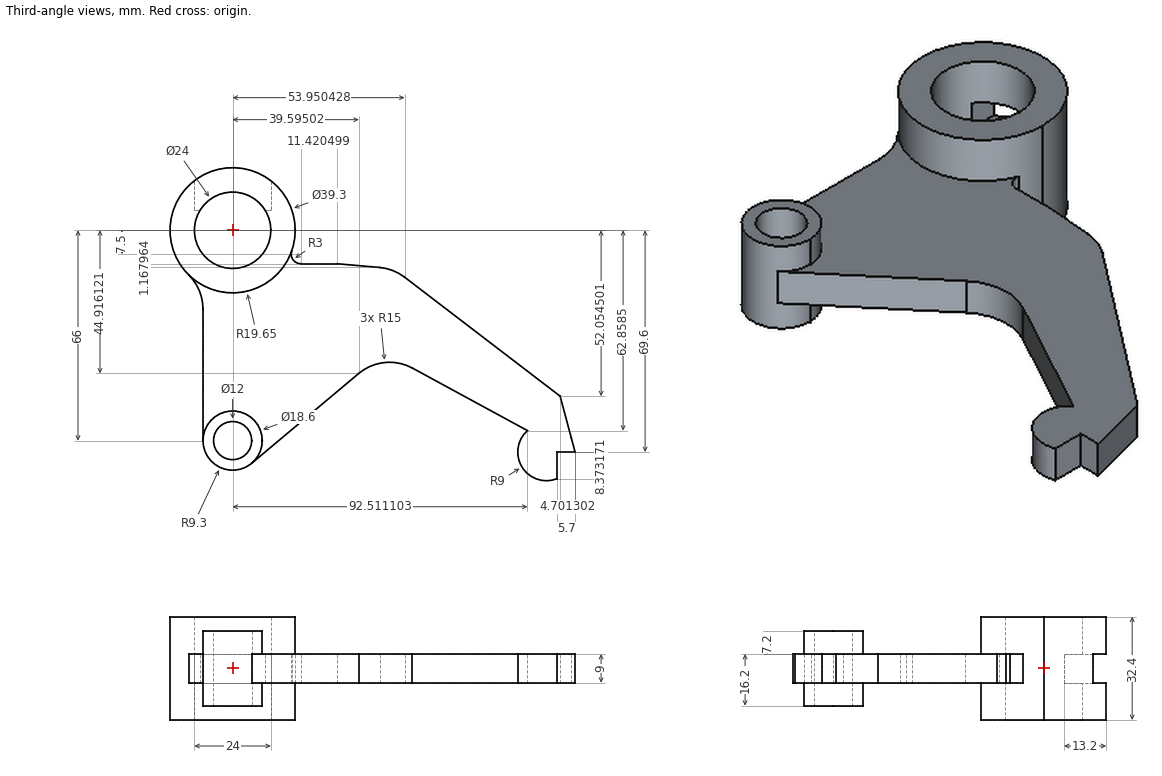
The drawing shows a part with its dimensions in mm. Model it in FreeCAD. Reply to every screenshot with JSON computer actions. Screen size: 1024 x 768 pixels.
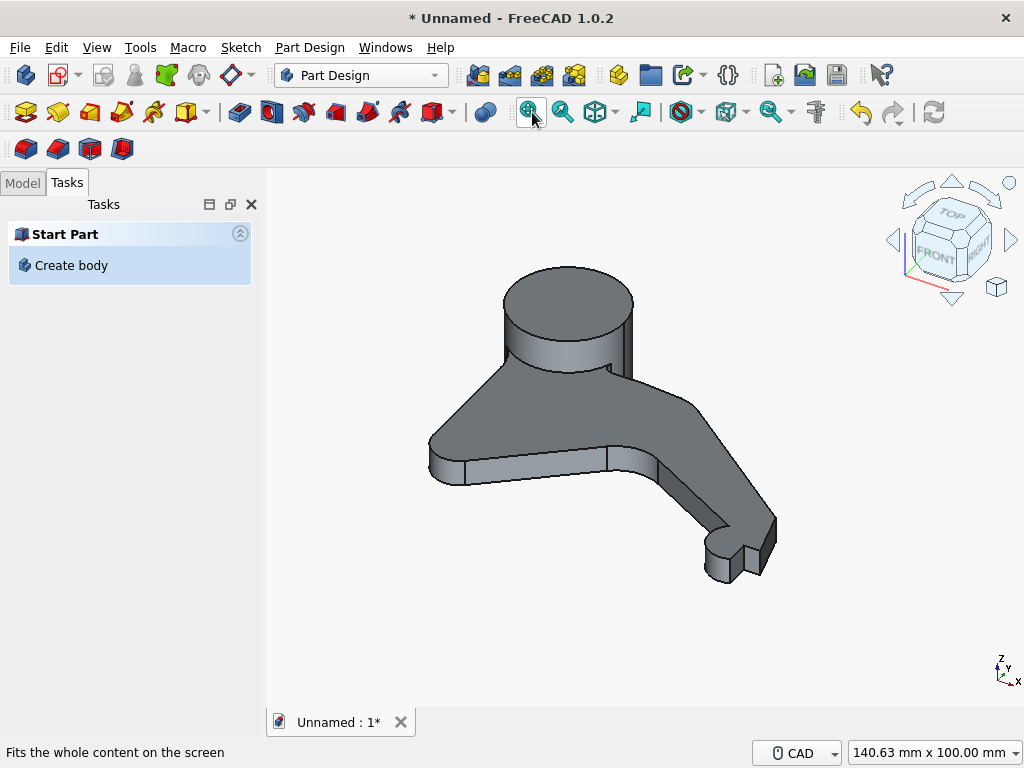
{"action": "left_click", "coordinate": [533, 416]}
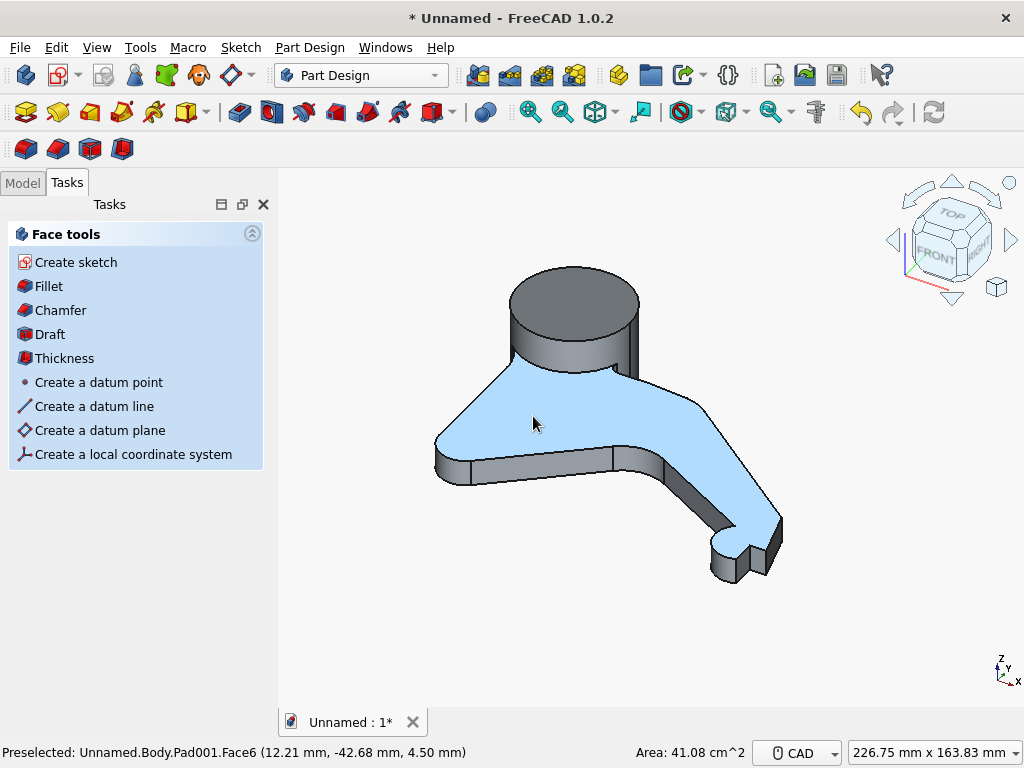
{"action": "left_click", "coordinate": [58, 76]}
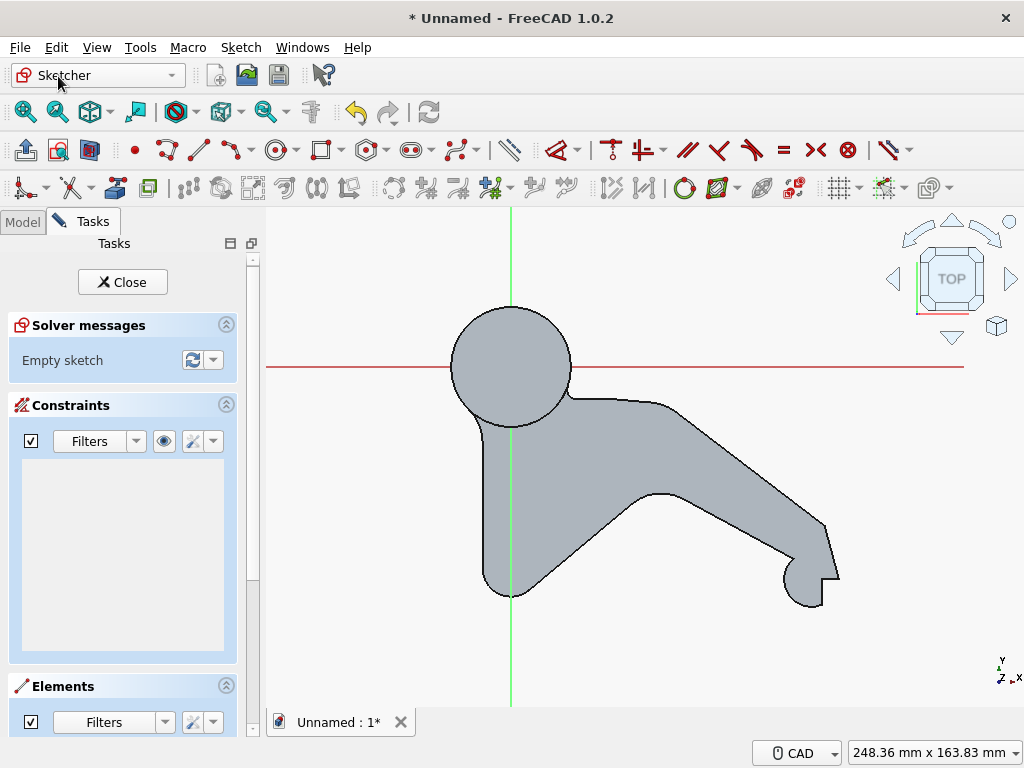
{"action": "left_click", "coordinate": [90, 150]}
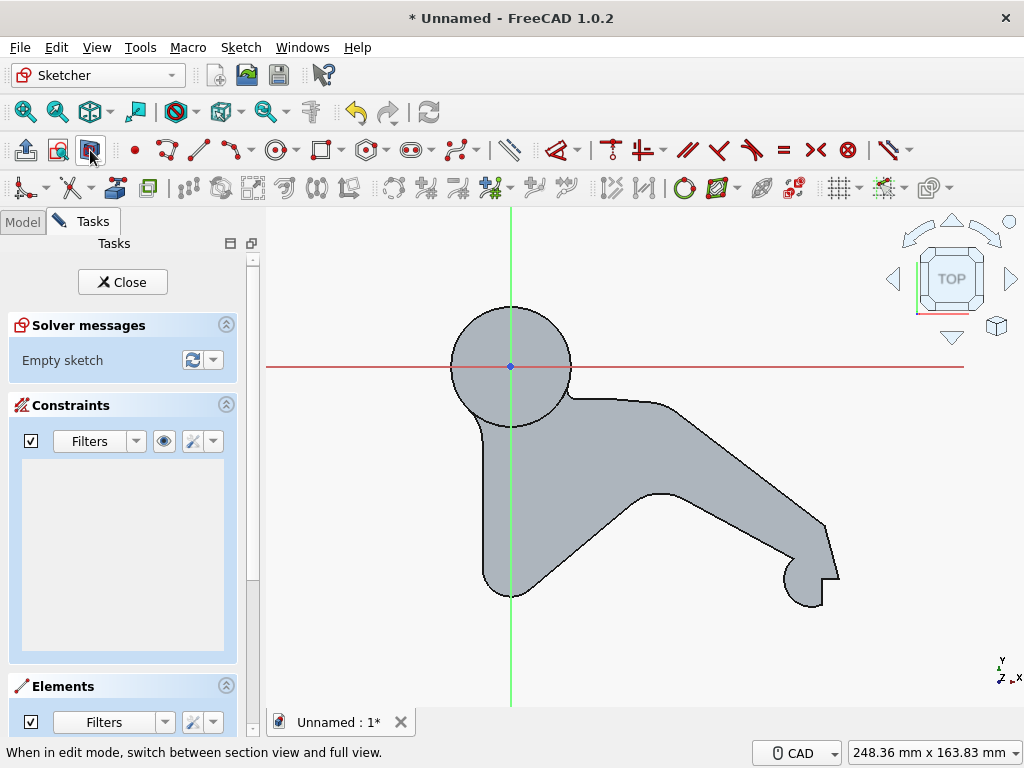
{"action": "scroll", "coordinate": [498, 590], "scroll_direction": "up", "scroll_amount": 9}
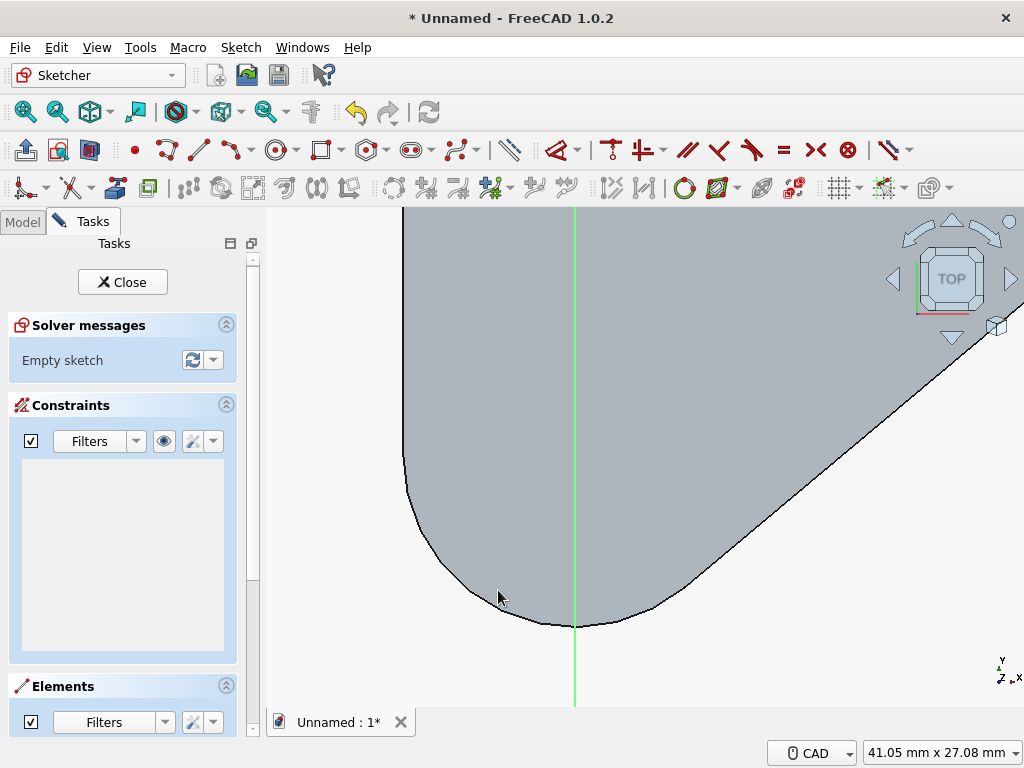
{"action": "left_click", "coordinate": [276, 150]}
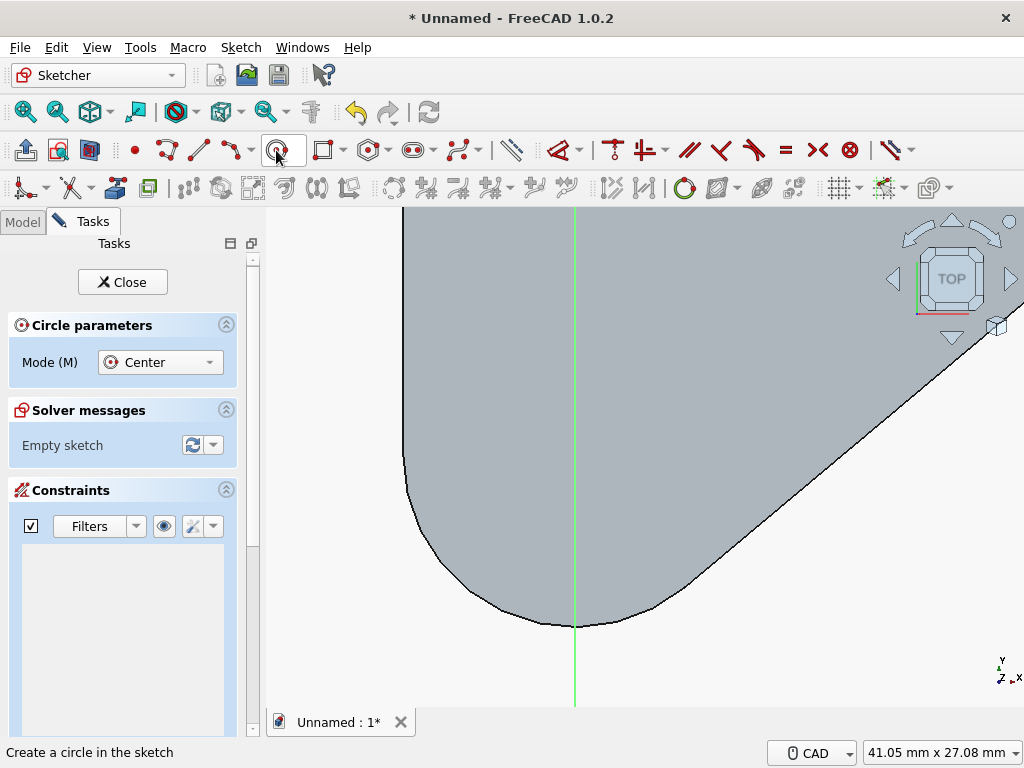
{"action": "left_click", "coordinate": [575, 455]}
{"action": "mouse_move", "coordinate": [696, 334]}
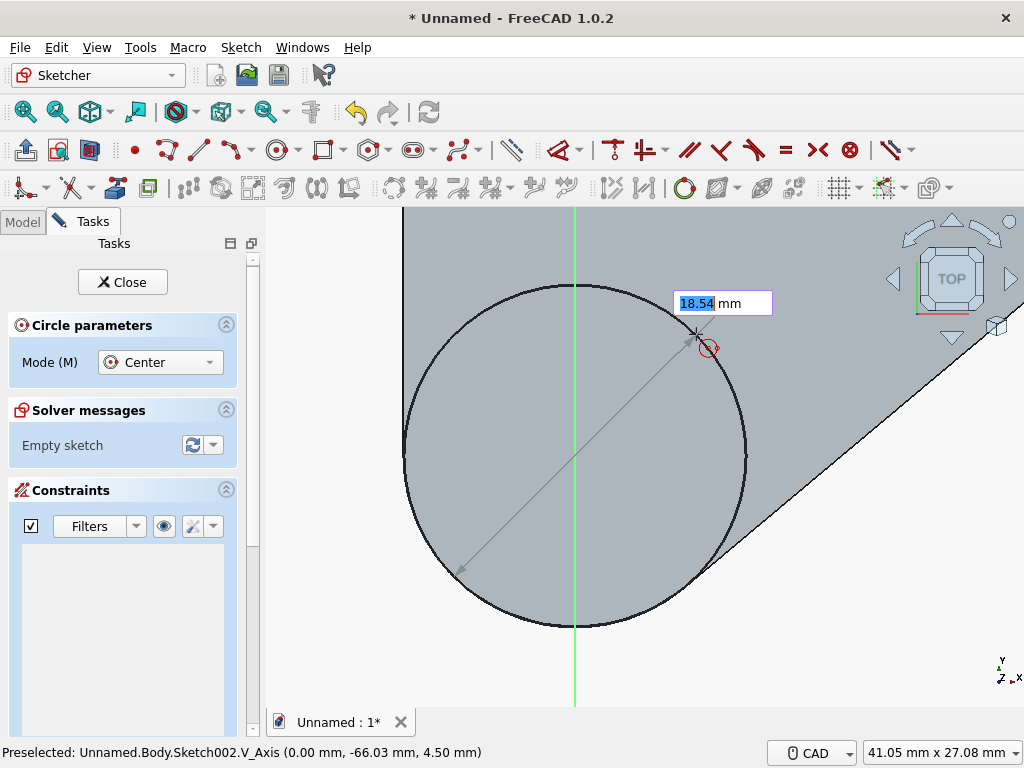
{"action": "type", "text": "18.6"}
{"action": "key", "text": "Return"}
{"action": "key", "text": "Escape"}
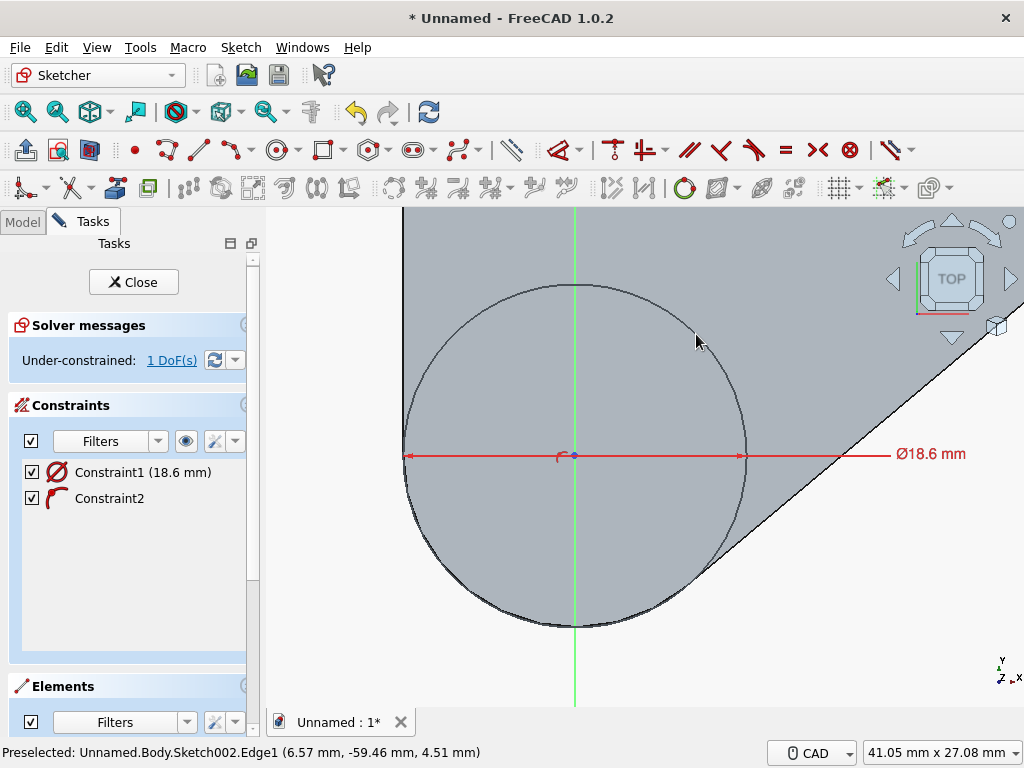
{"action": "left_click", "coordinate": [558, 150]}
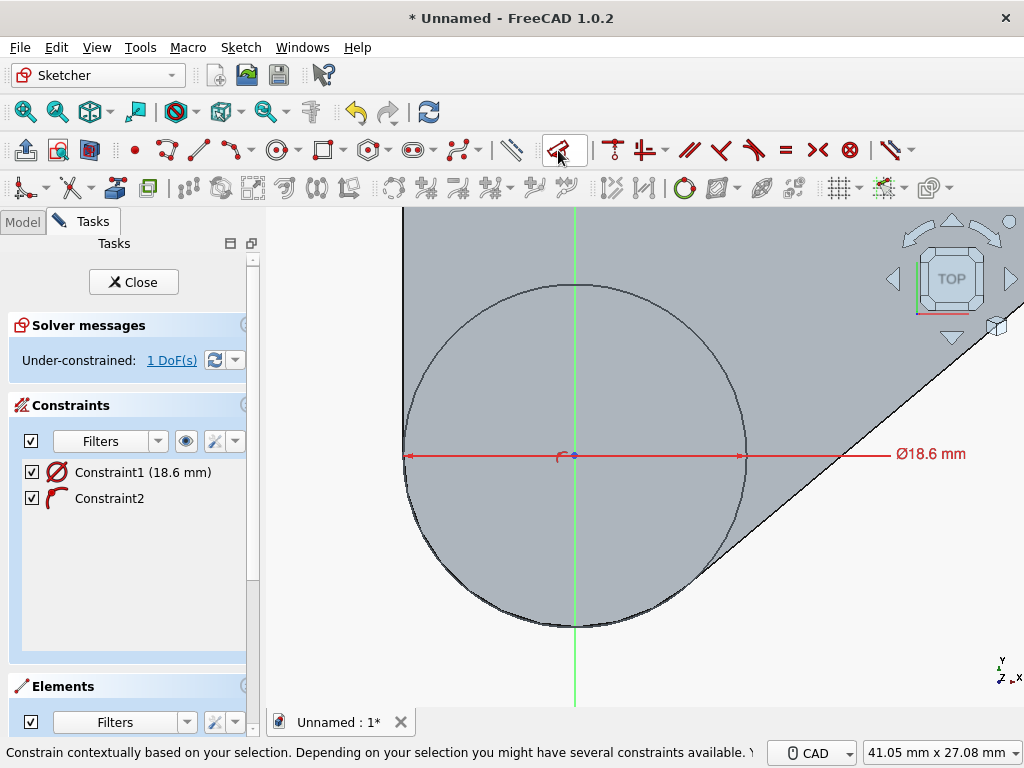
{"action": "left_click", "coordinate": [575, 456]}
{"action": "left_click", "coordinate": [609, 346]}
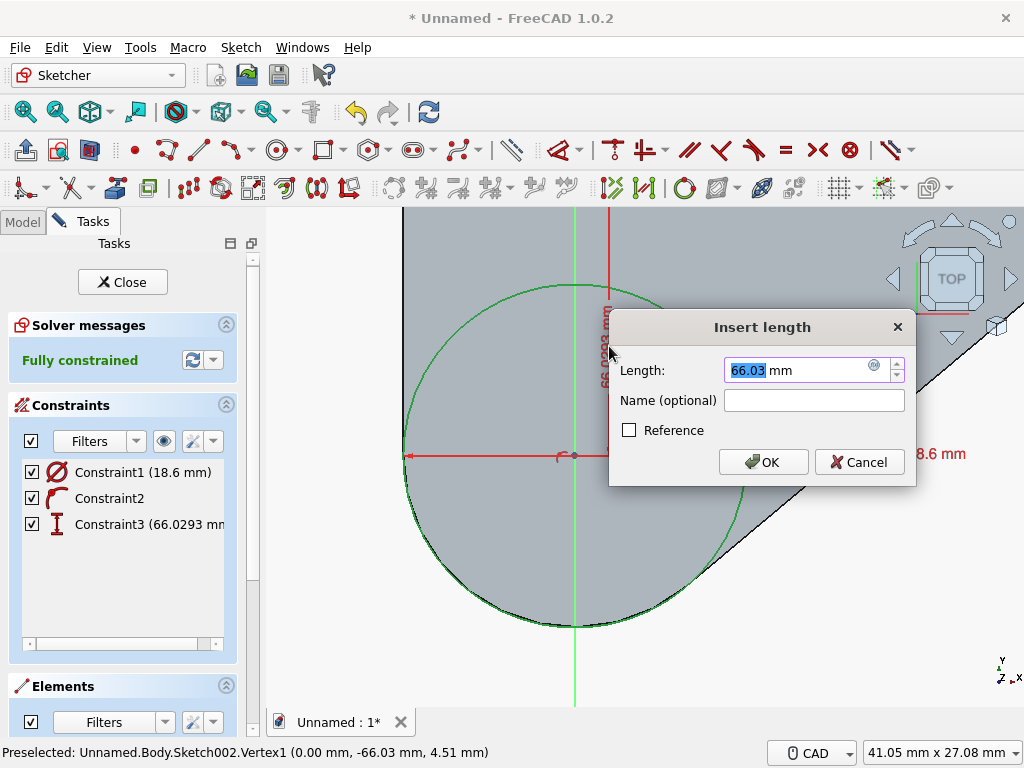
{"action": "type", "text": "66"}
{"action": "key", "text": "Return"}
{"action": "key", "text": "Escape"}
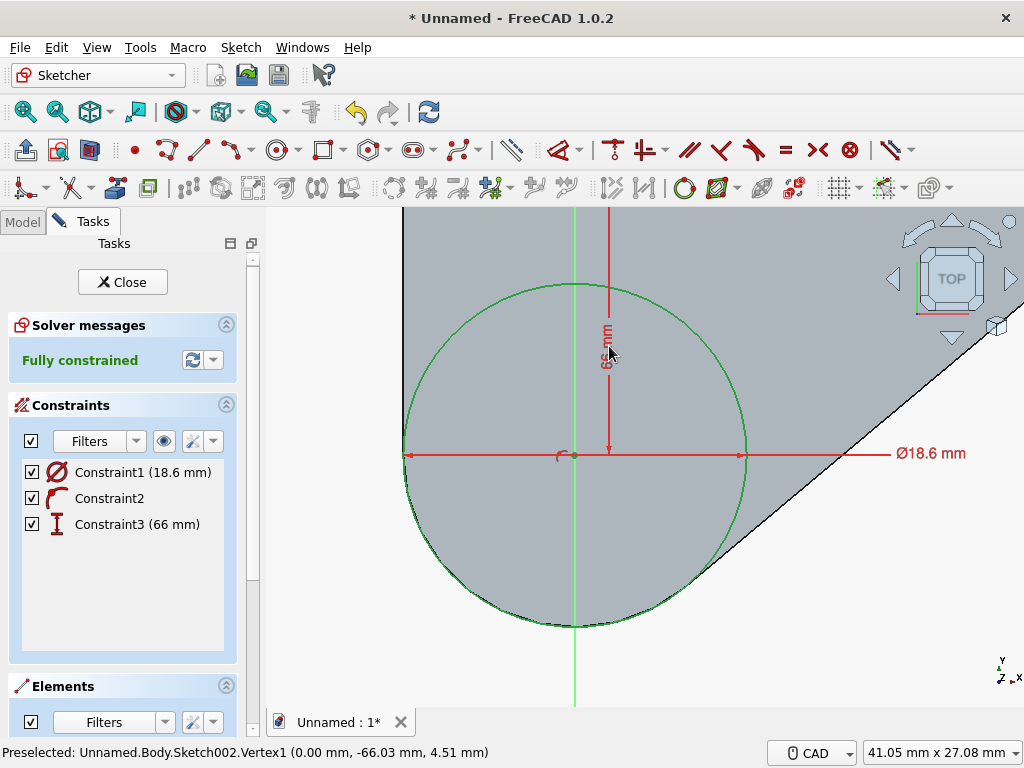
{"action": "left_click", "coordinate": [123, 282]}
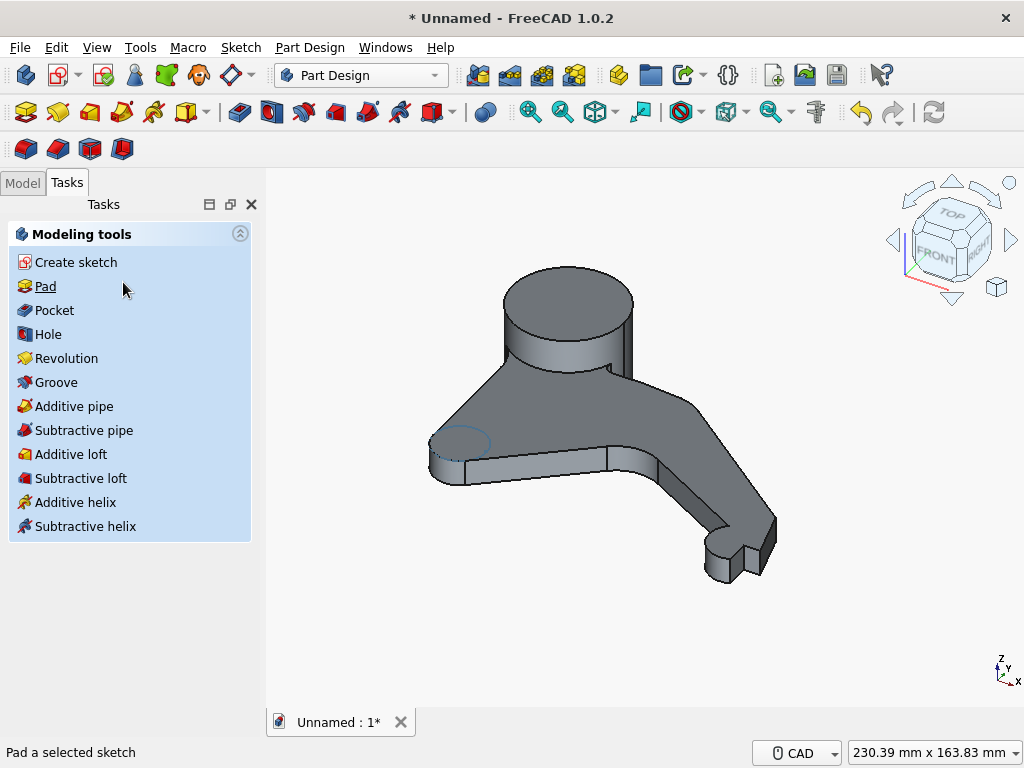
{"action": "left_click", "coordinate": [26, 112]}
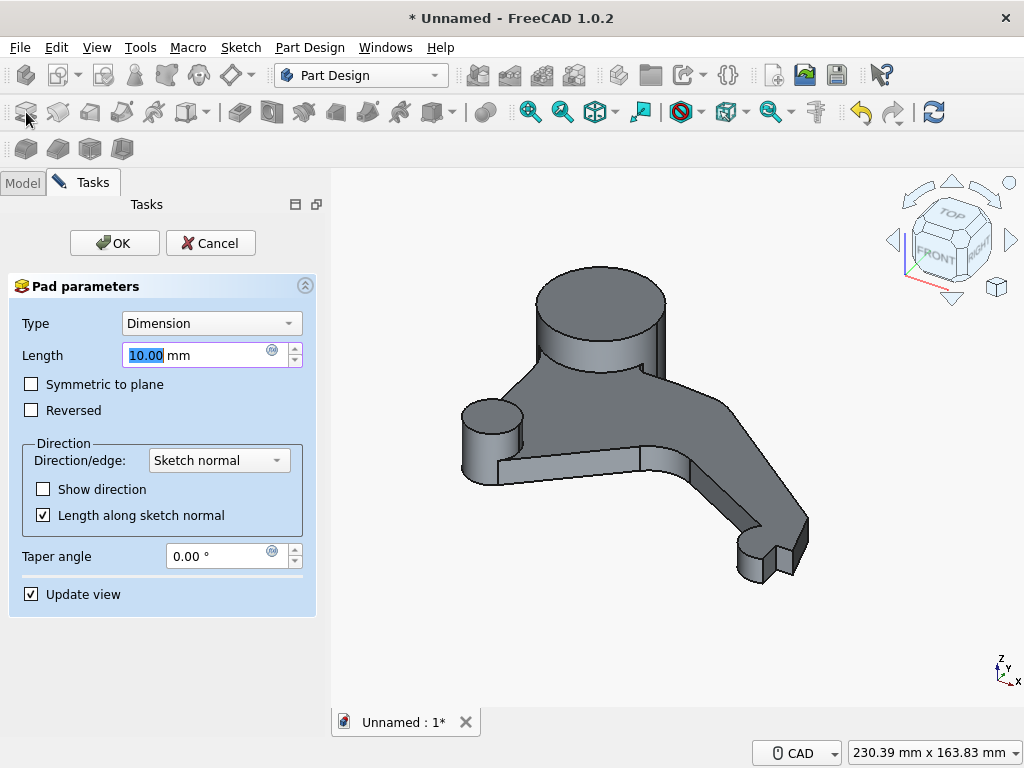
{"action": "left_click", "coordinate": [212, 324]}